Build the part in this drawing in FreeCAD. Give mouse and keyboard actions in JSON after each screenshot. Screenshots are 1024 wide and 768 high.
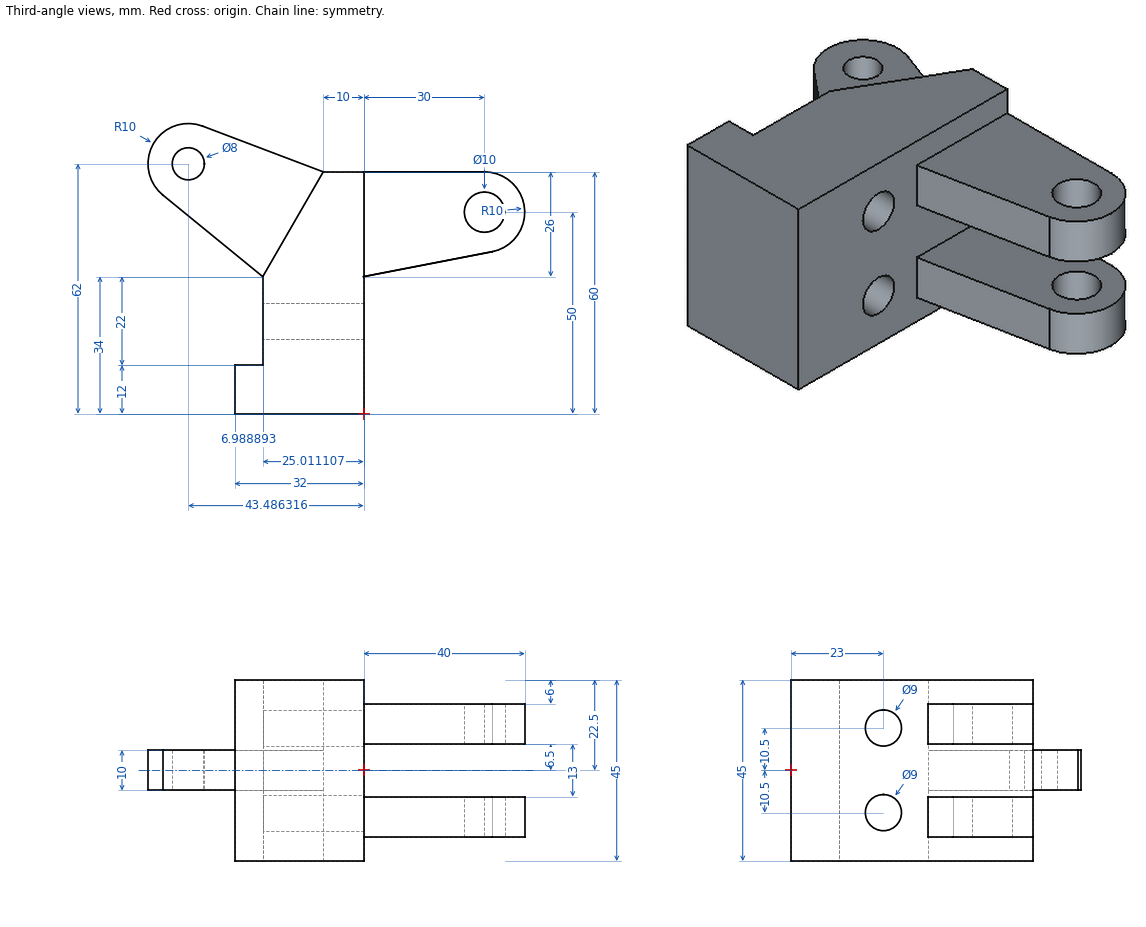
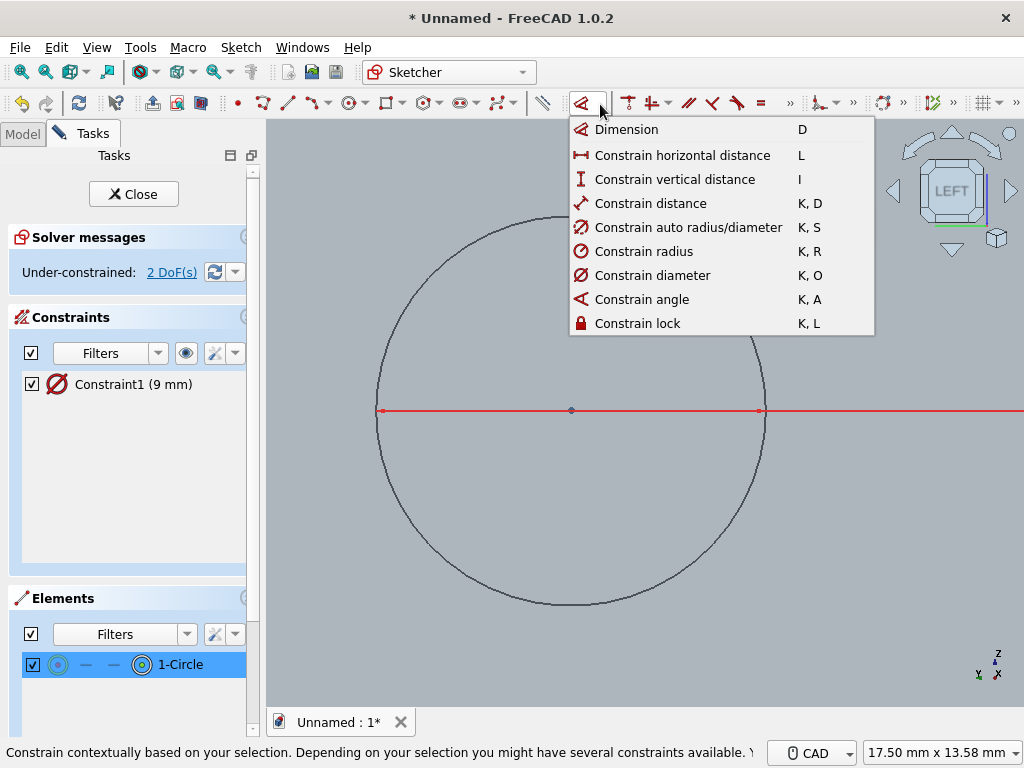
{"action": "left_click", "coordinate": [722, 155]}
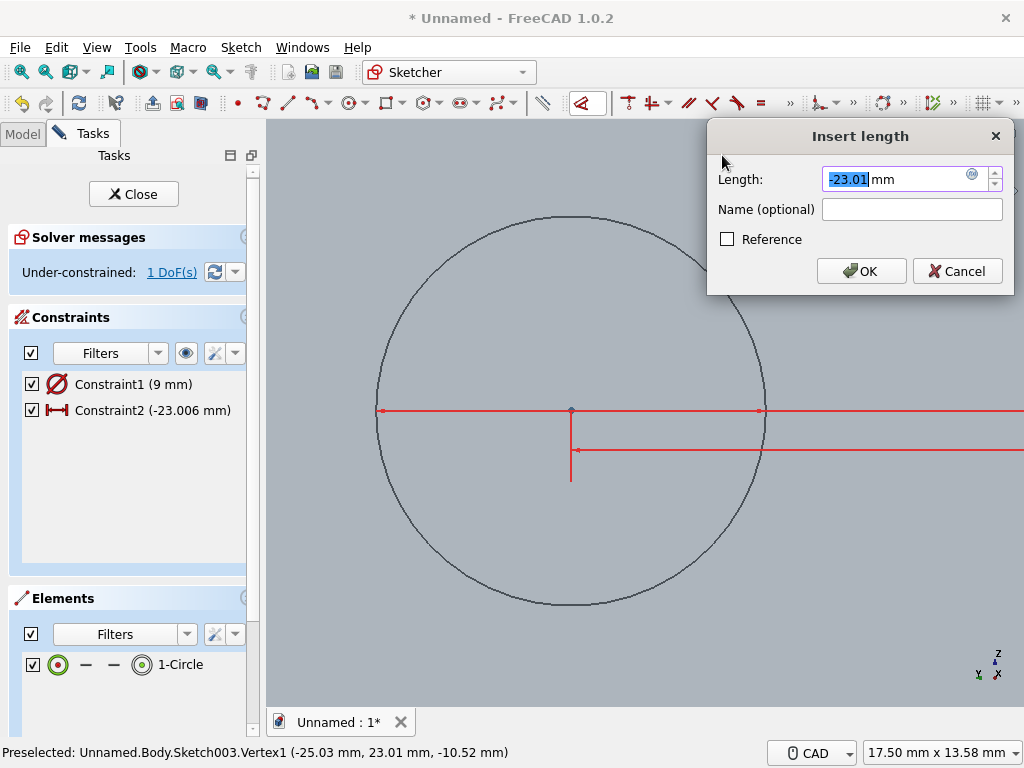
{"action": "type", "text": "-23"}
{"action": "key", "text": "Return"}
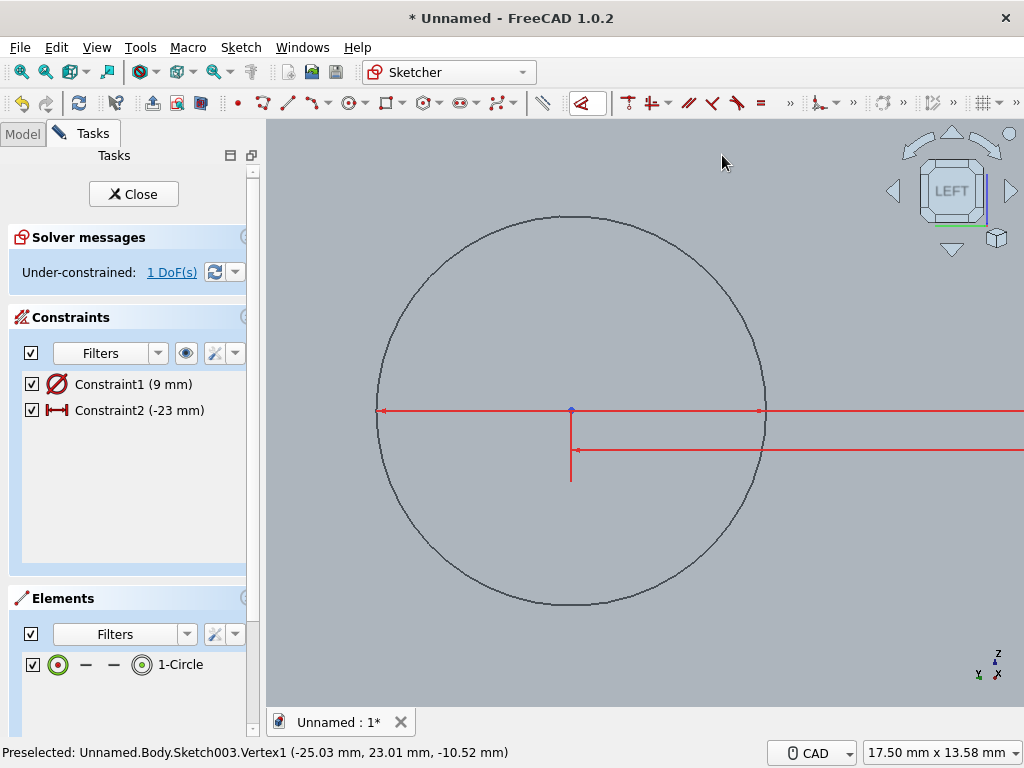
{"action": "left_click", "coordinate": [571, 411]}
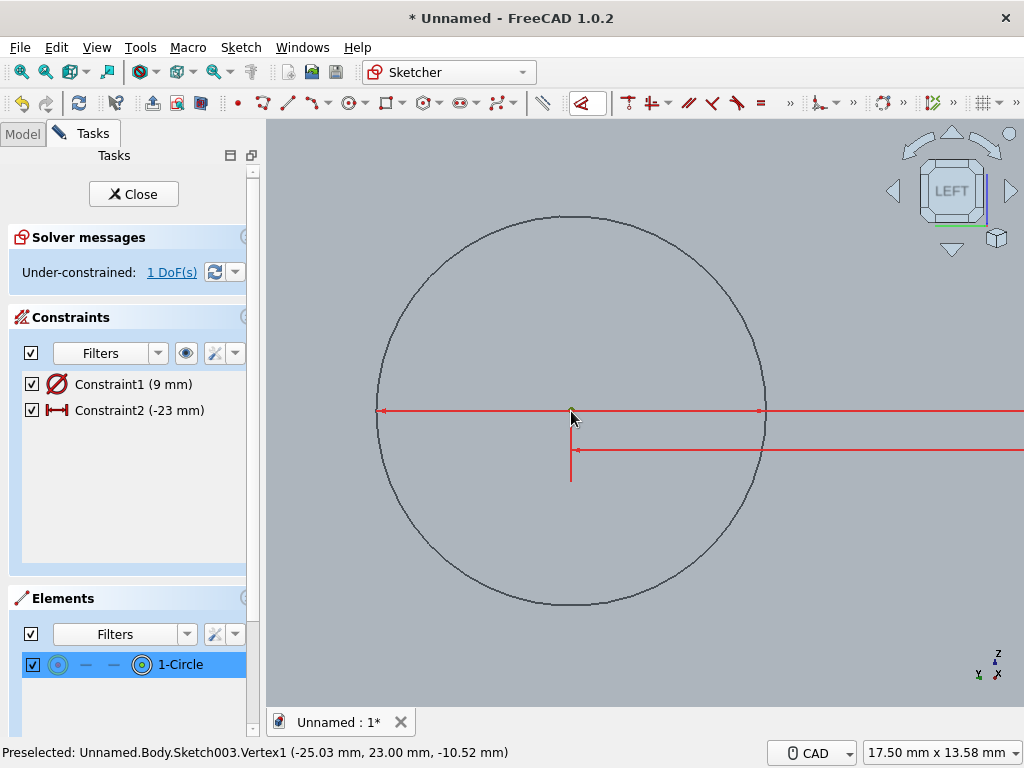
{"action": "key", "text": "i"}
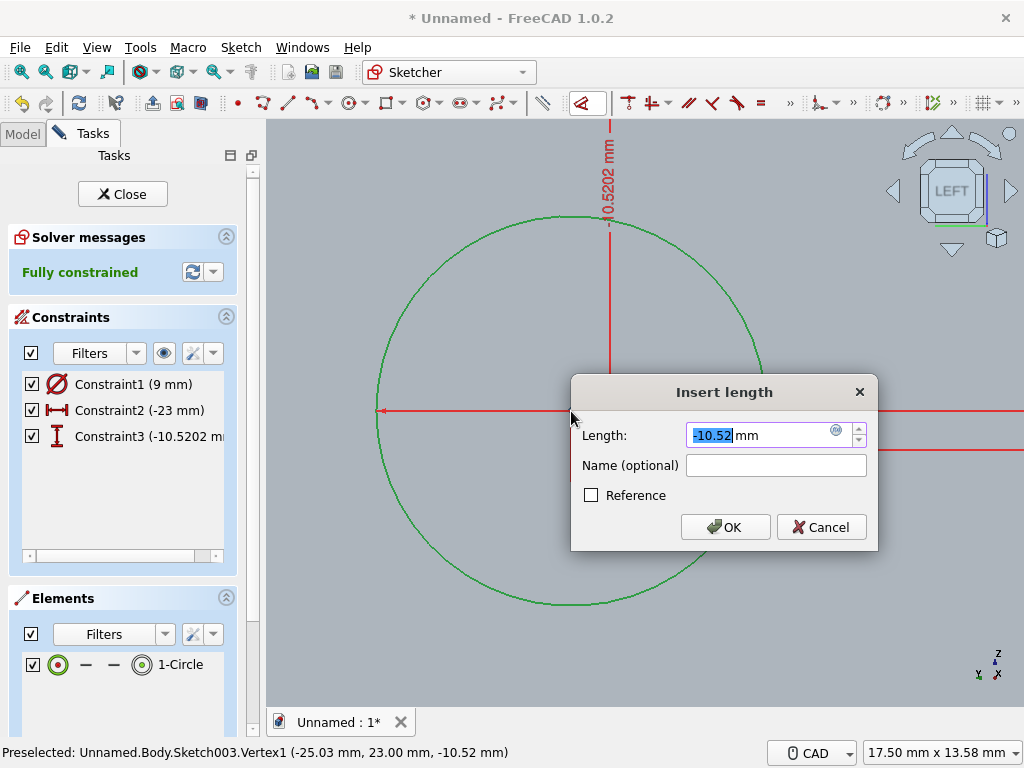
{"action": "type", "text": "-10.5"}
{"action": "key", "text": "Return"}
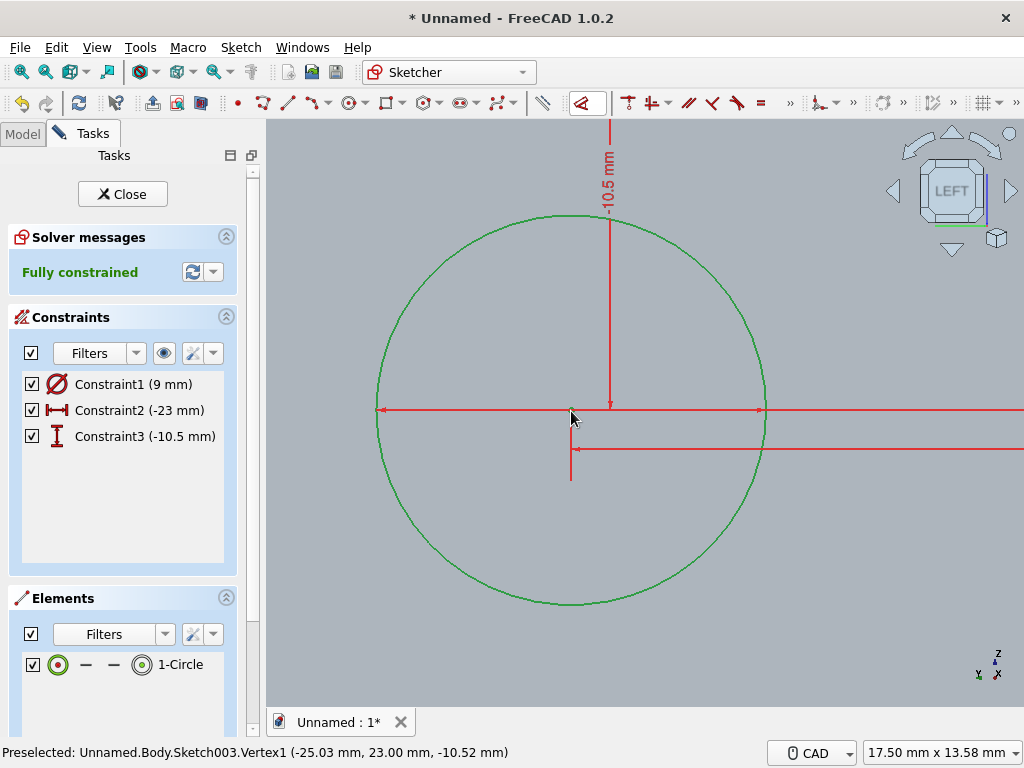
{"action": "left_click", "coordinate": [123, 194]}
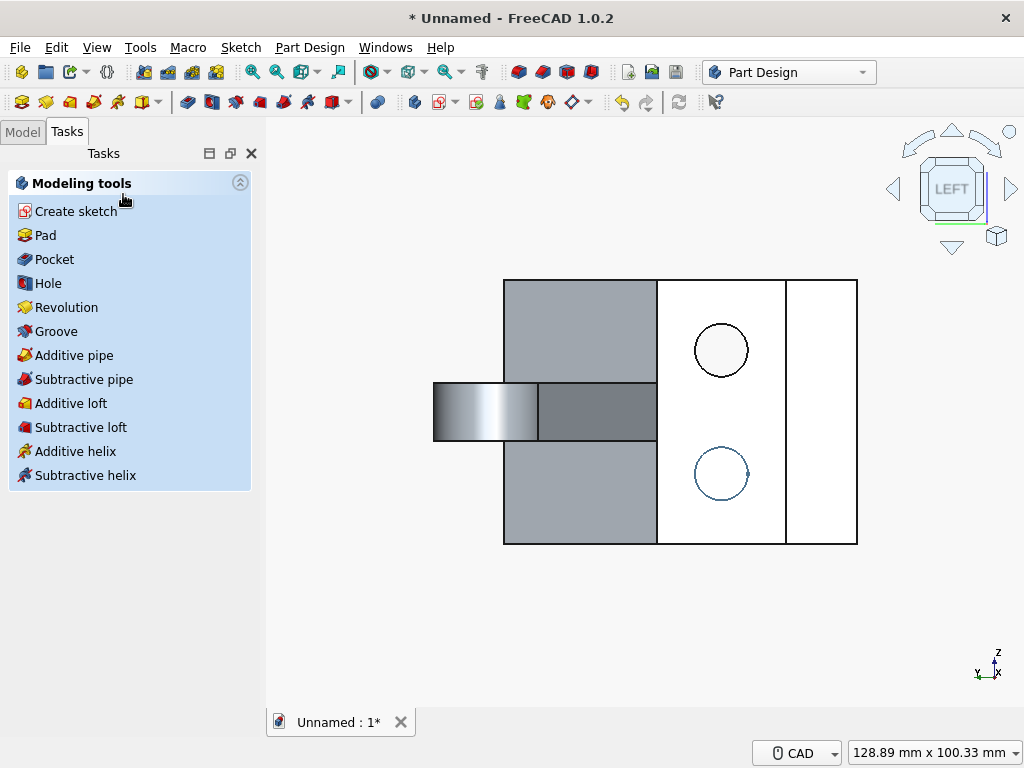
{"action": "left_click", "coordinate": [188, 102]}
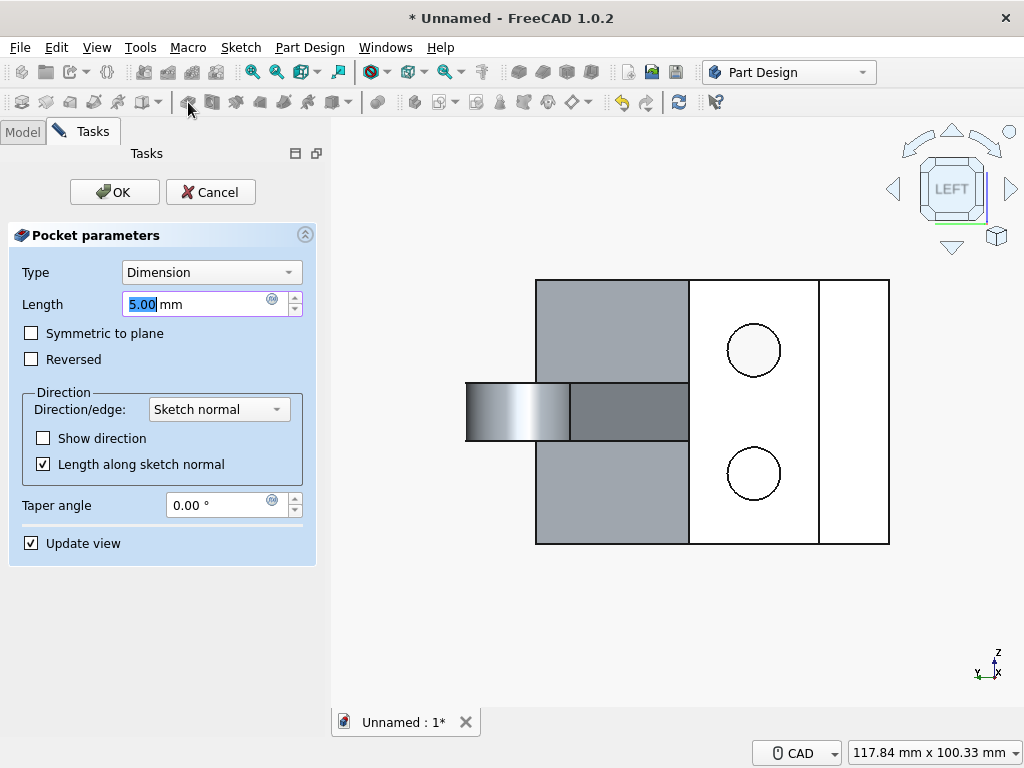
{"action": "left_click", "coordinate": [212, 272]}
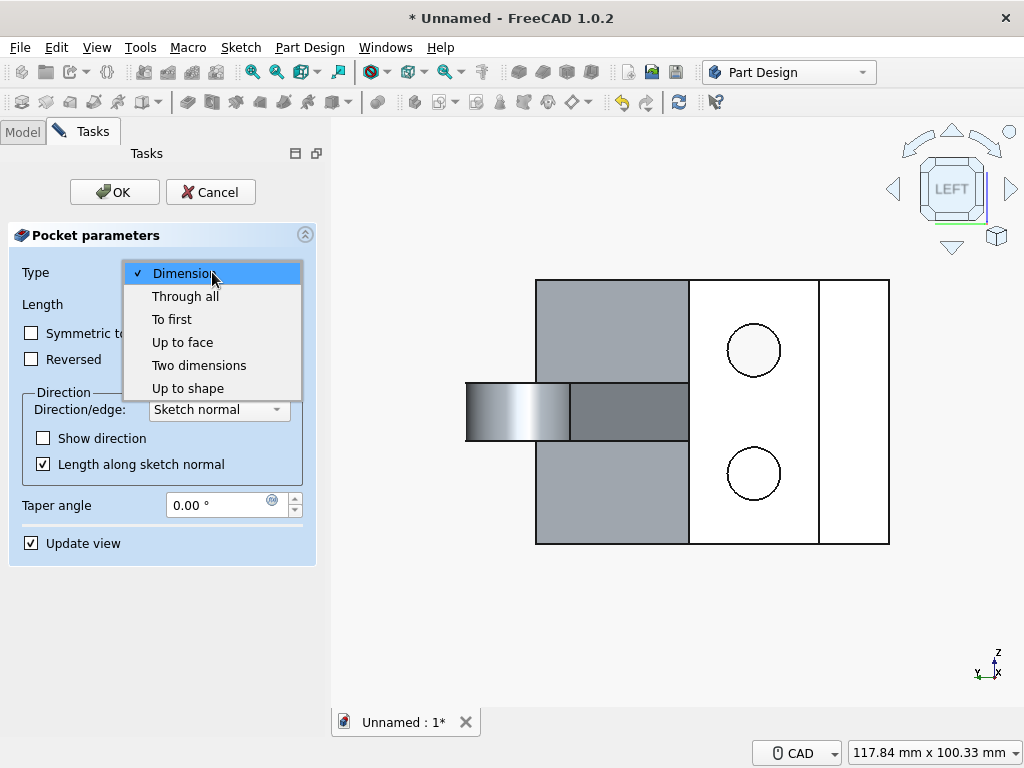
{"action": "left_click", "coordinate": [212, 320]}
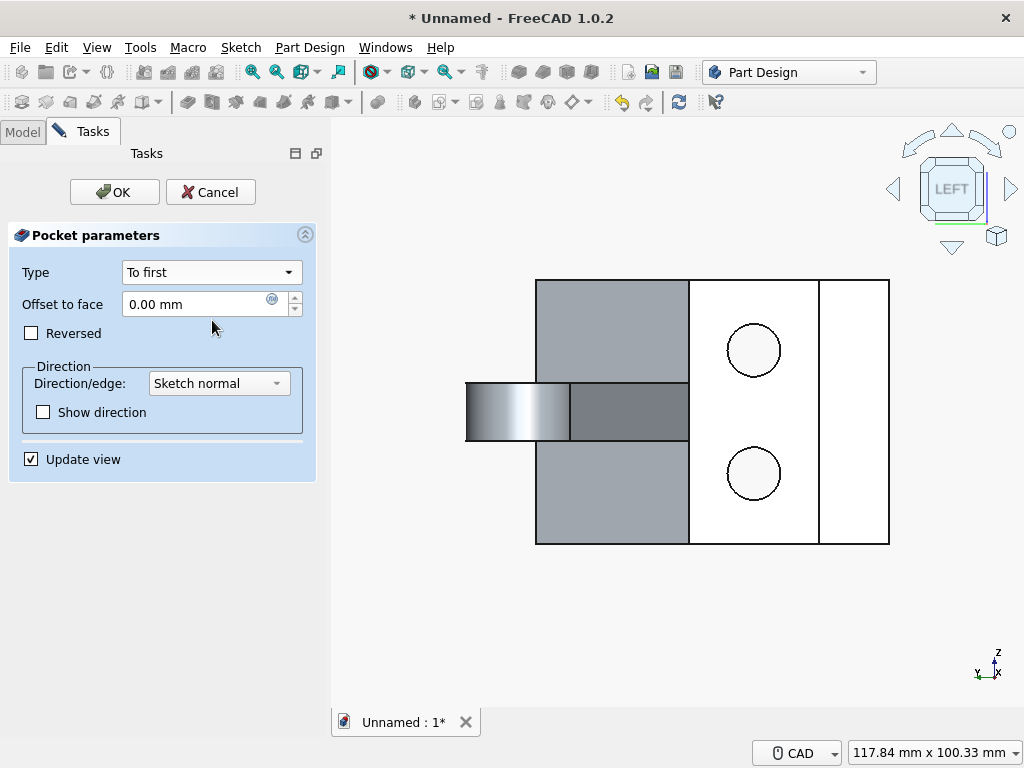
{"action": "left_click", "coordinate": [115, 192]}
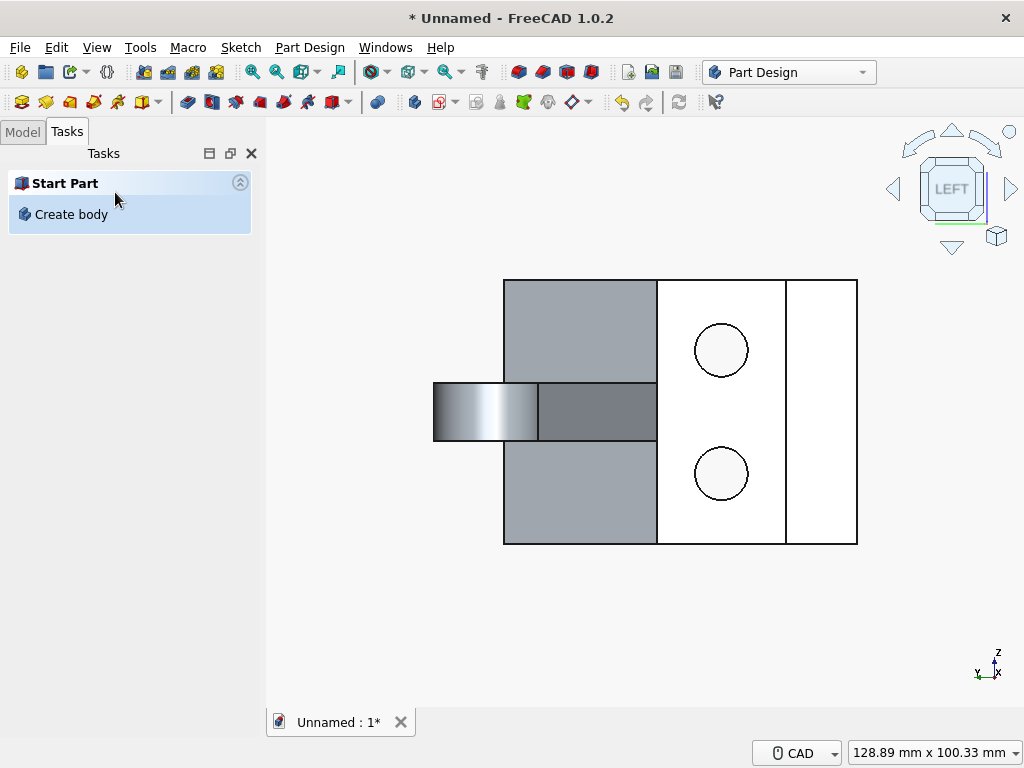
{"action": "key", "text": "0"}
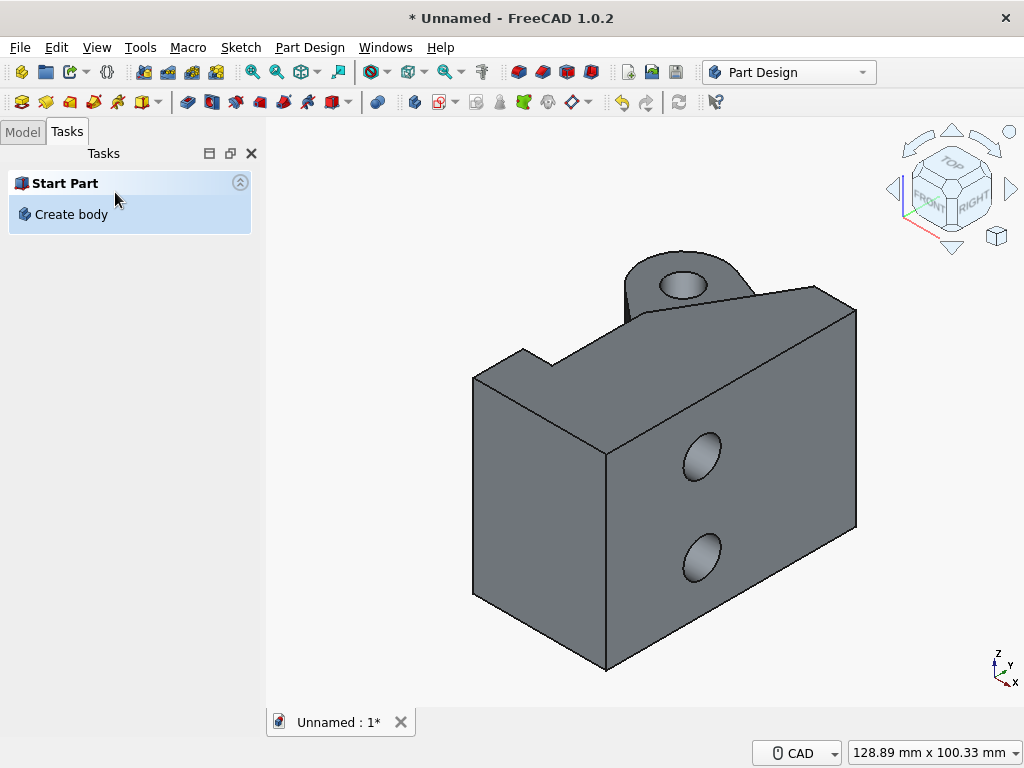
{"action": "left_click", "coordinate": [684, 354]}